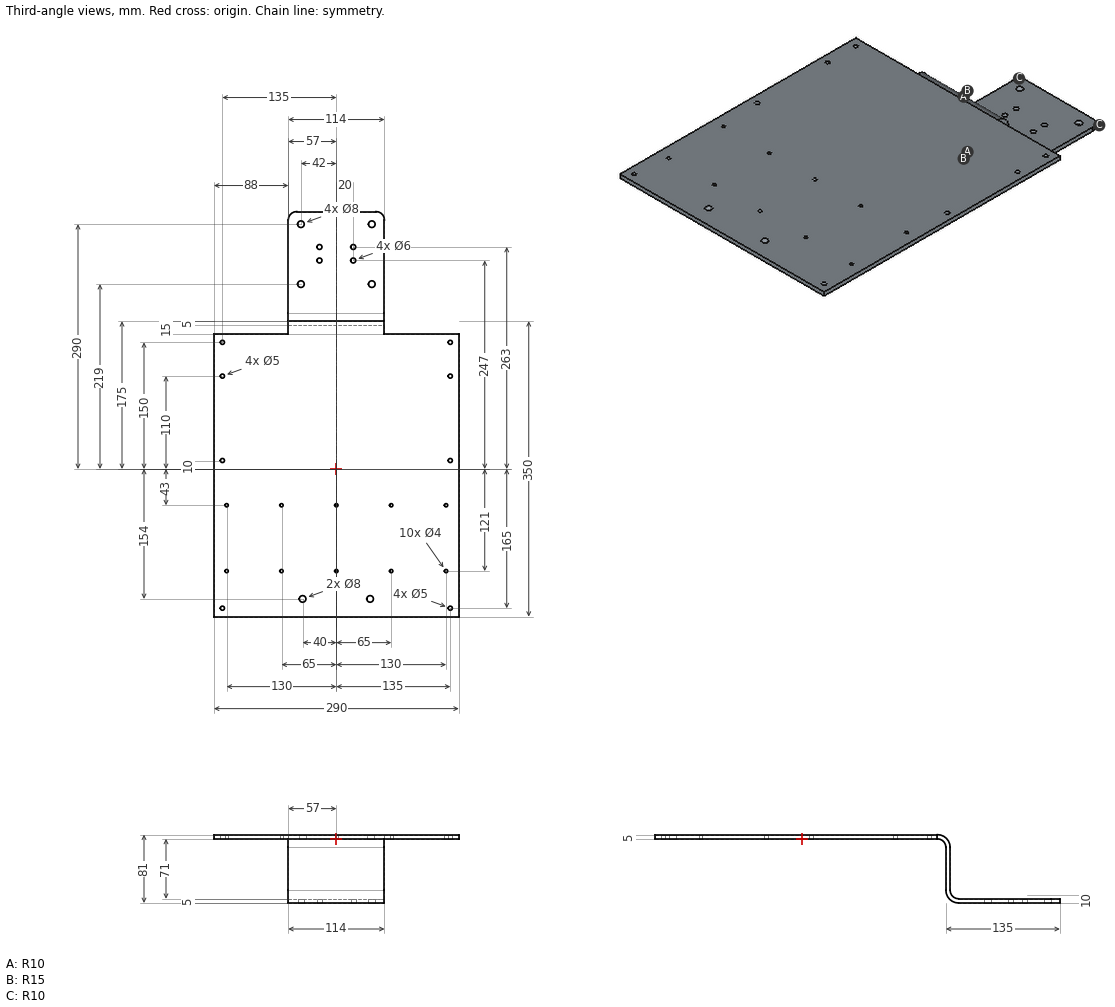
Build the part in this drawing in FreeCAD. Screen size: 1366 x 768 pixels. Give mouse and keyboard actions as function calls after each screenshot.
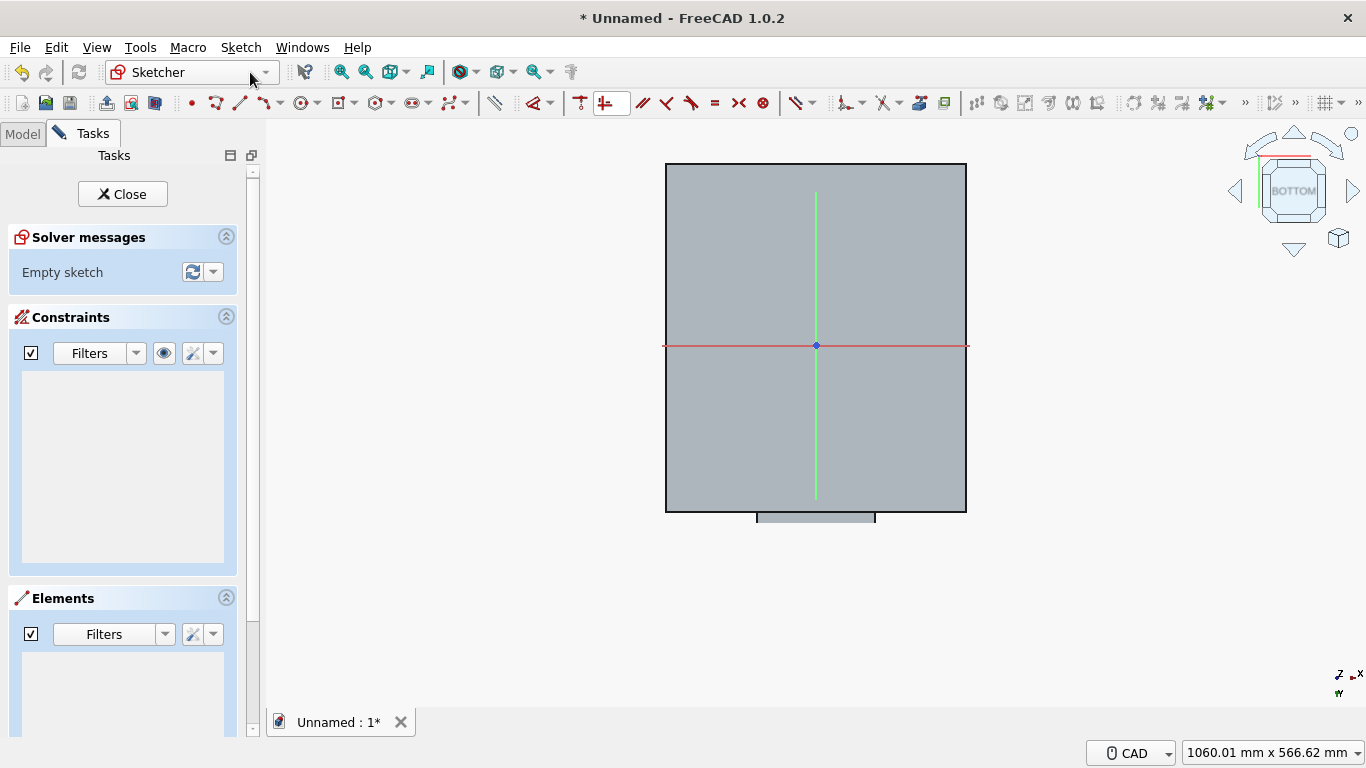
scroll(872, 175, up, 4)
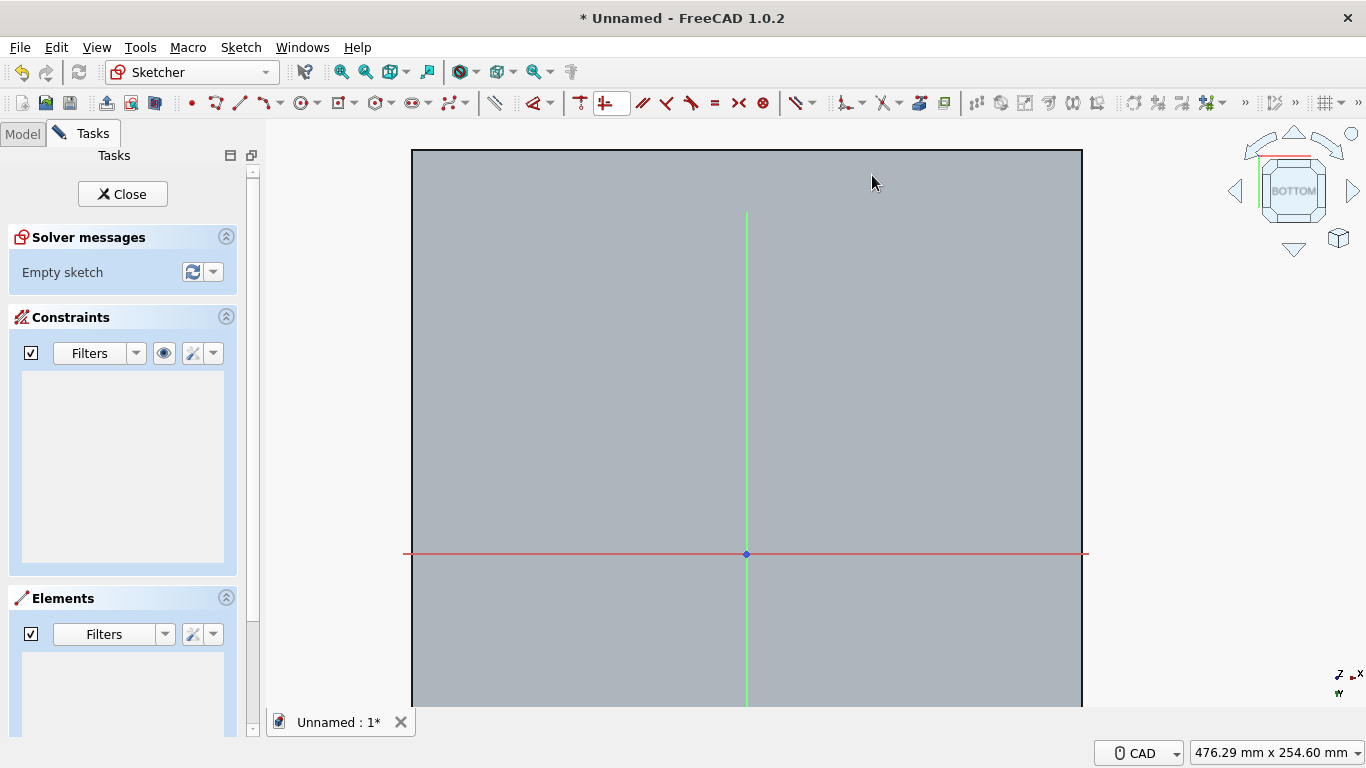
click(302, 104)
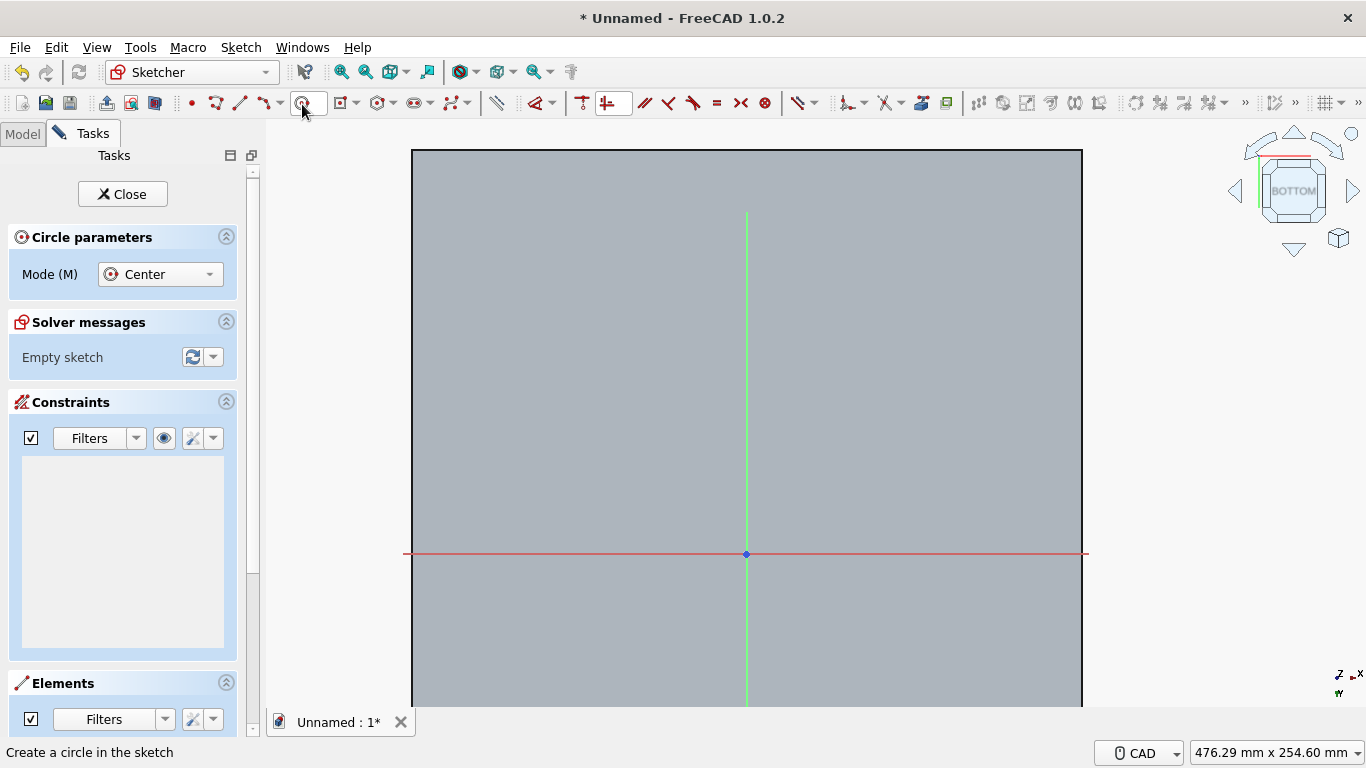
scroll(1047, 275, up, 8)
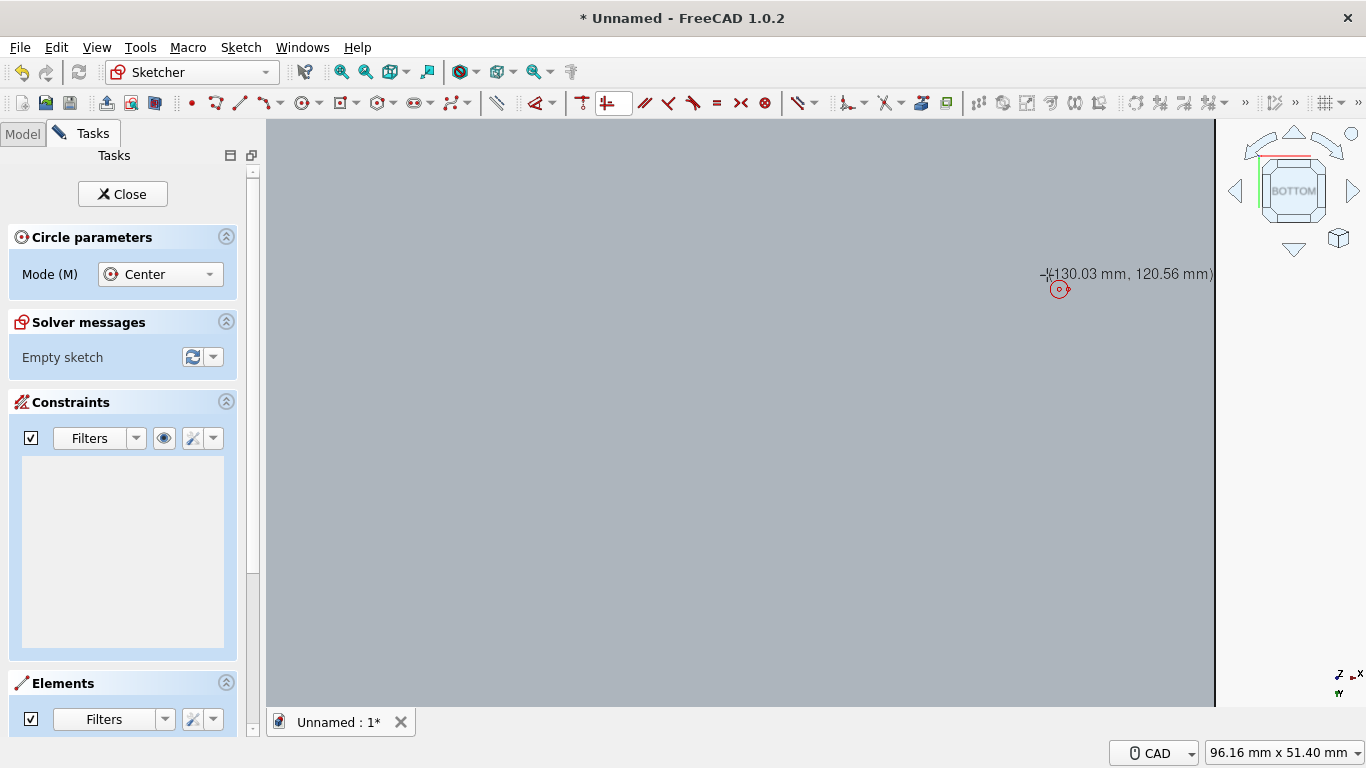
scroll(1049, 276, down, 8)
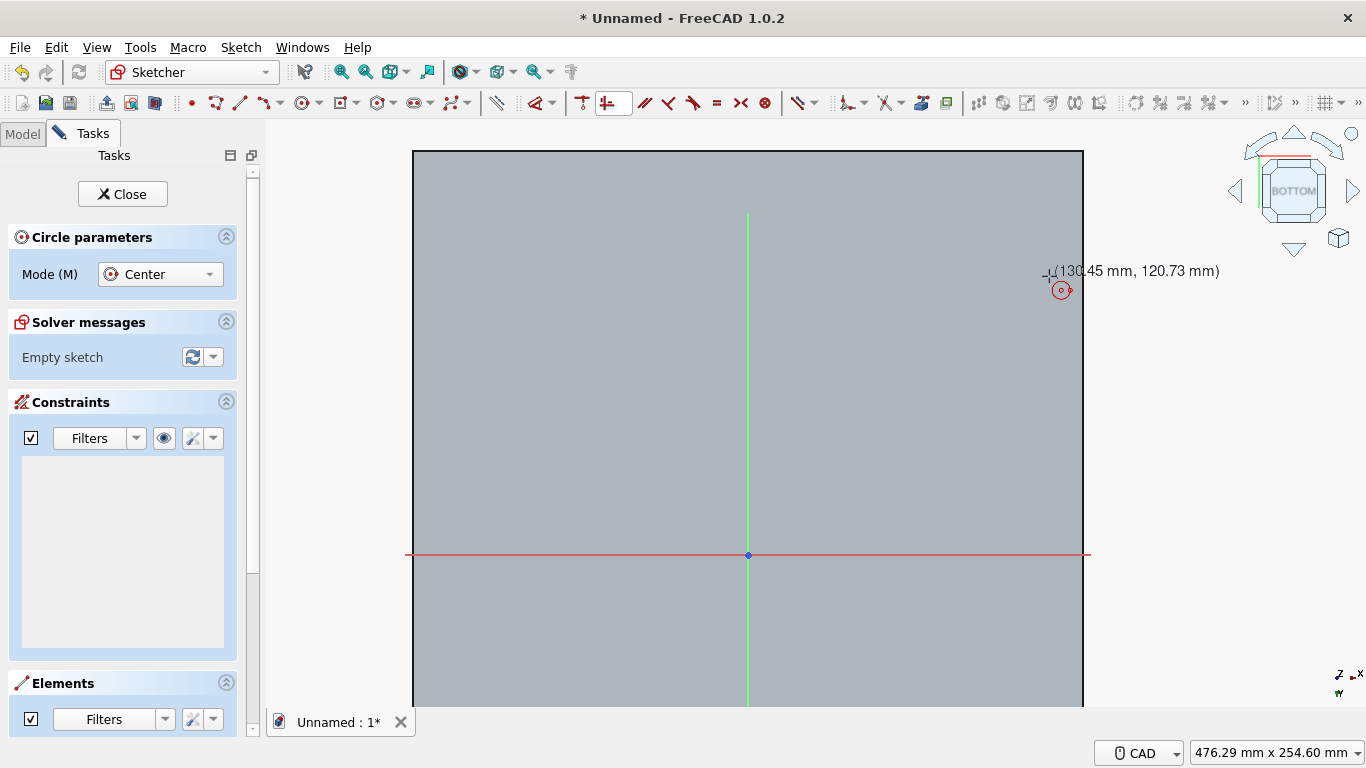
click(1049, 276)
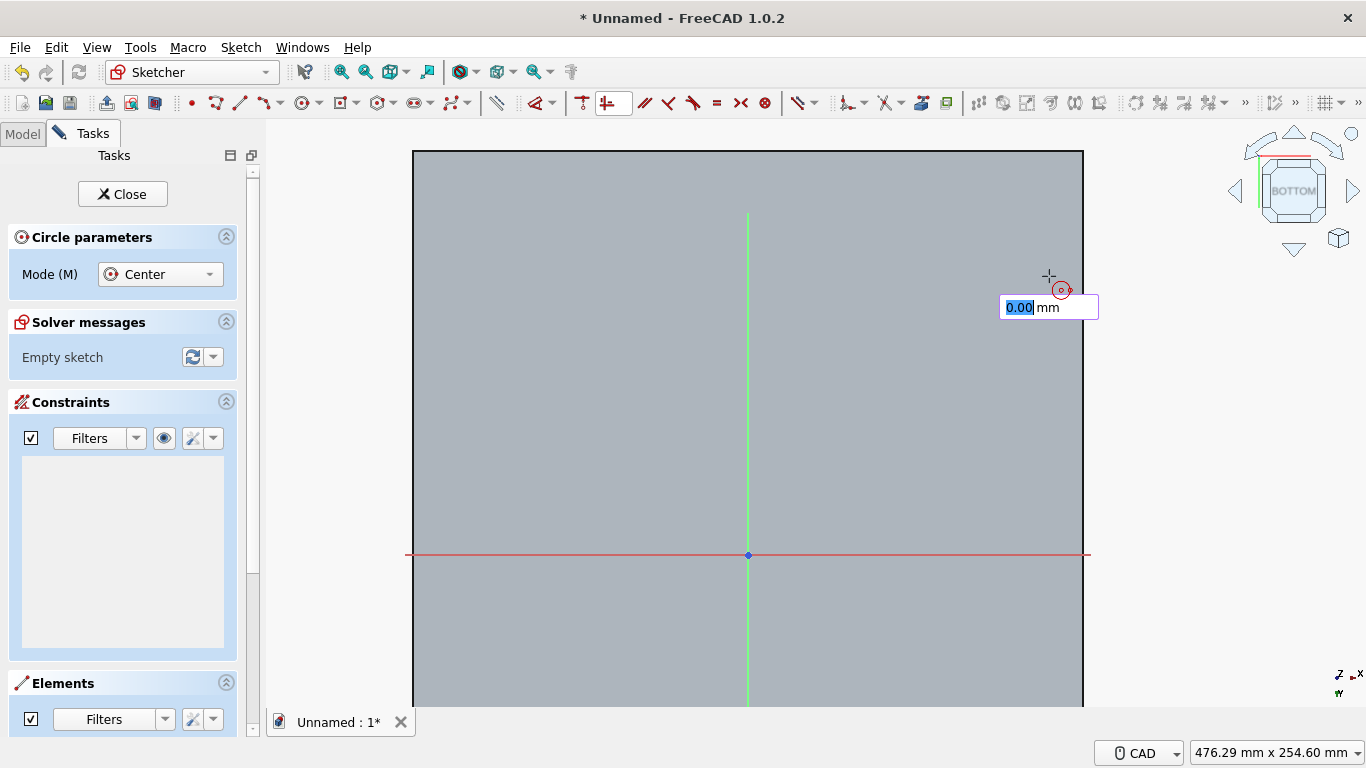
scroll(1052, 273, up, 7)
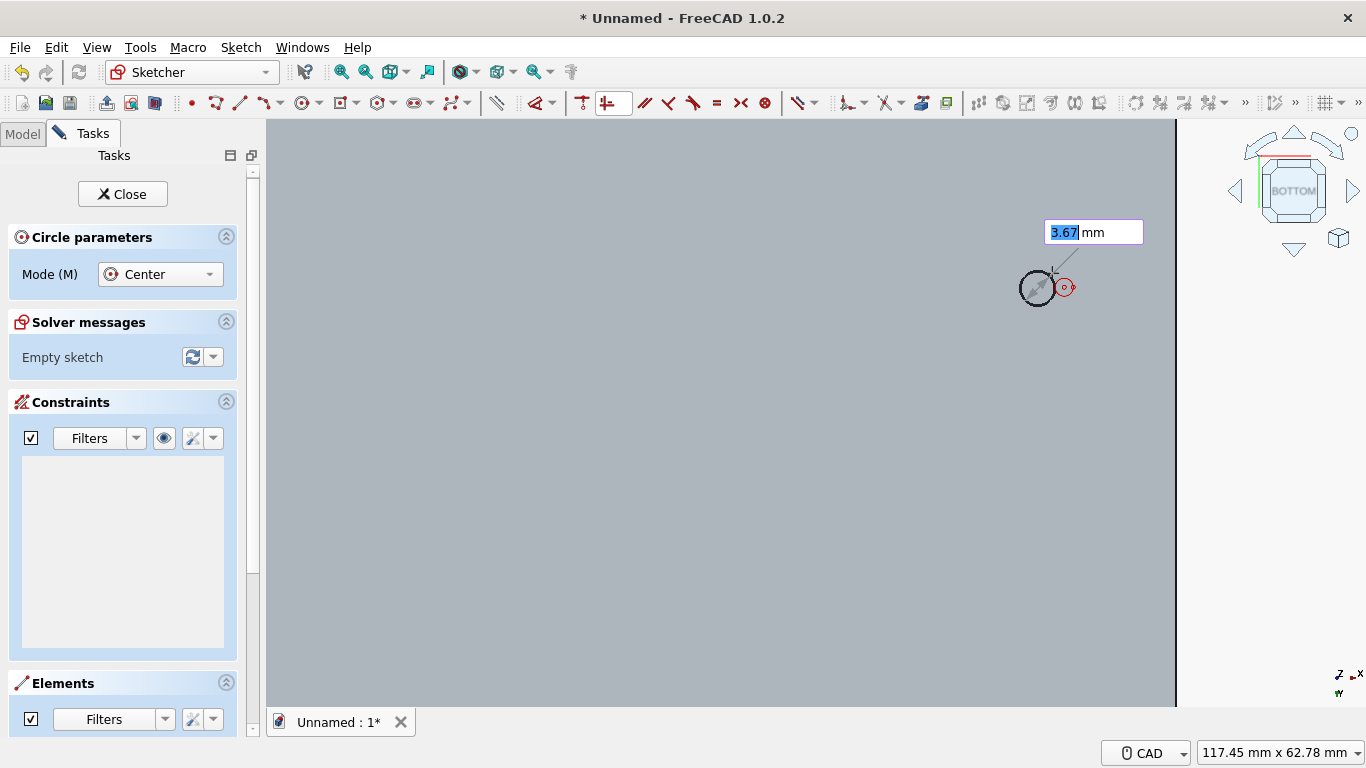
click(1049, 270)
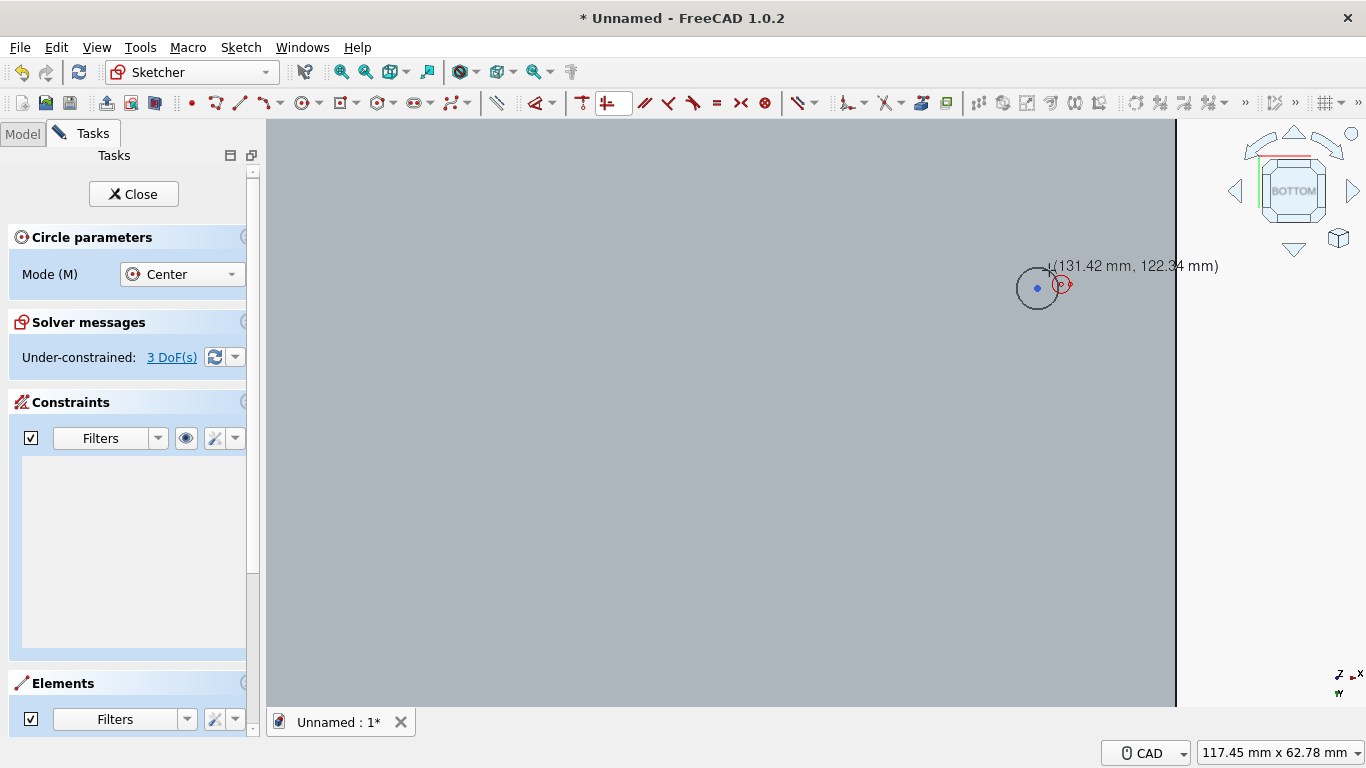
scroll(1052, 273, down, 7)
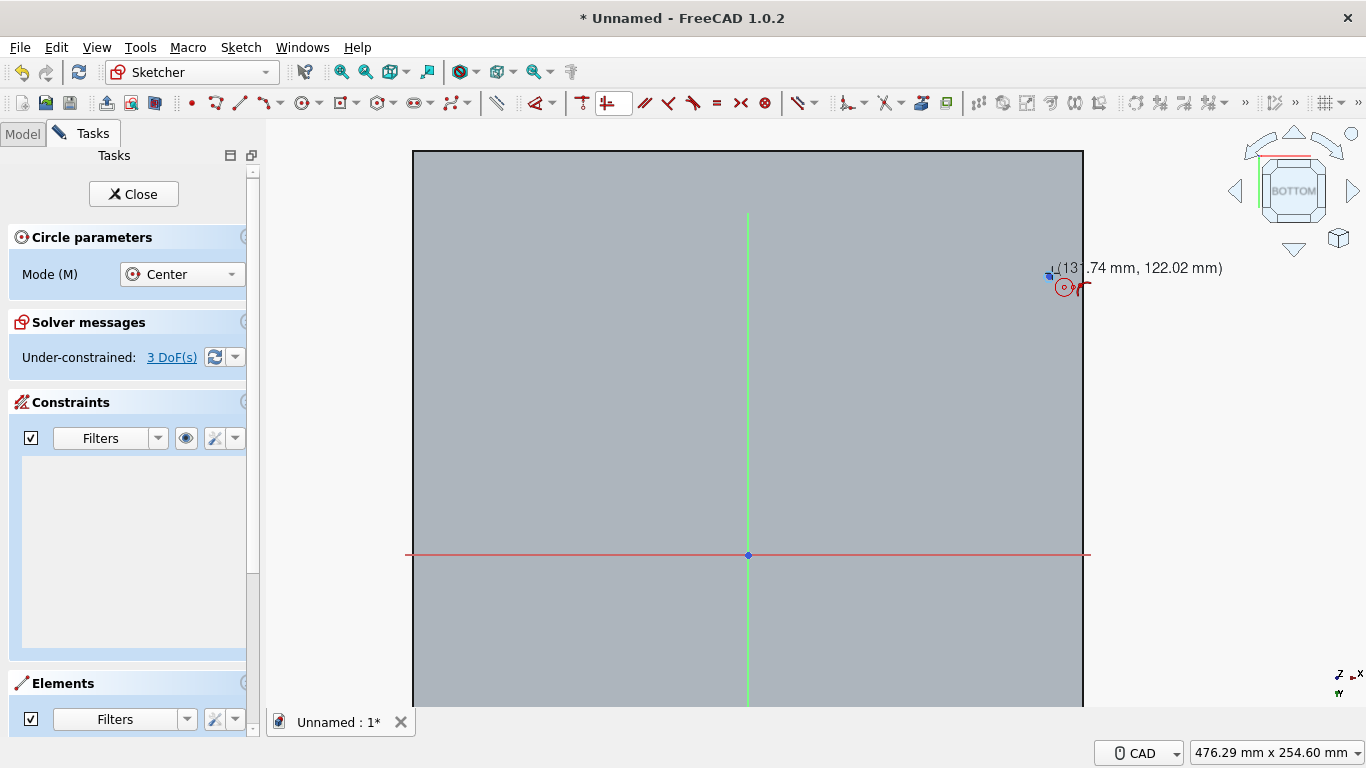
click(898, 276)